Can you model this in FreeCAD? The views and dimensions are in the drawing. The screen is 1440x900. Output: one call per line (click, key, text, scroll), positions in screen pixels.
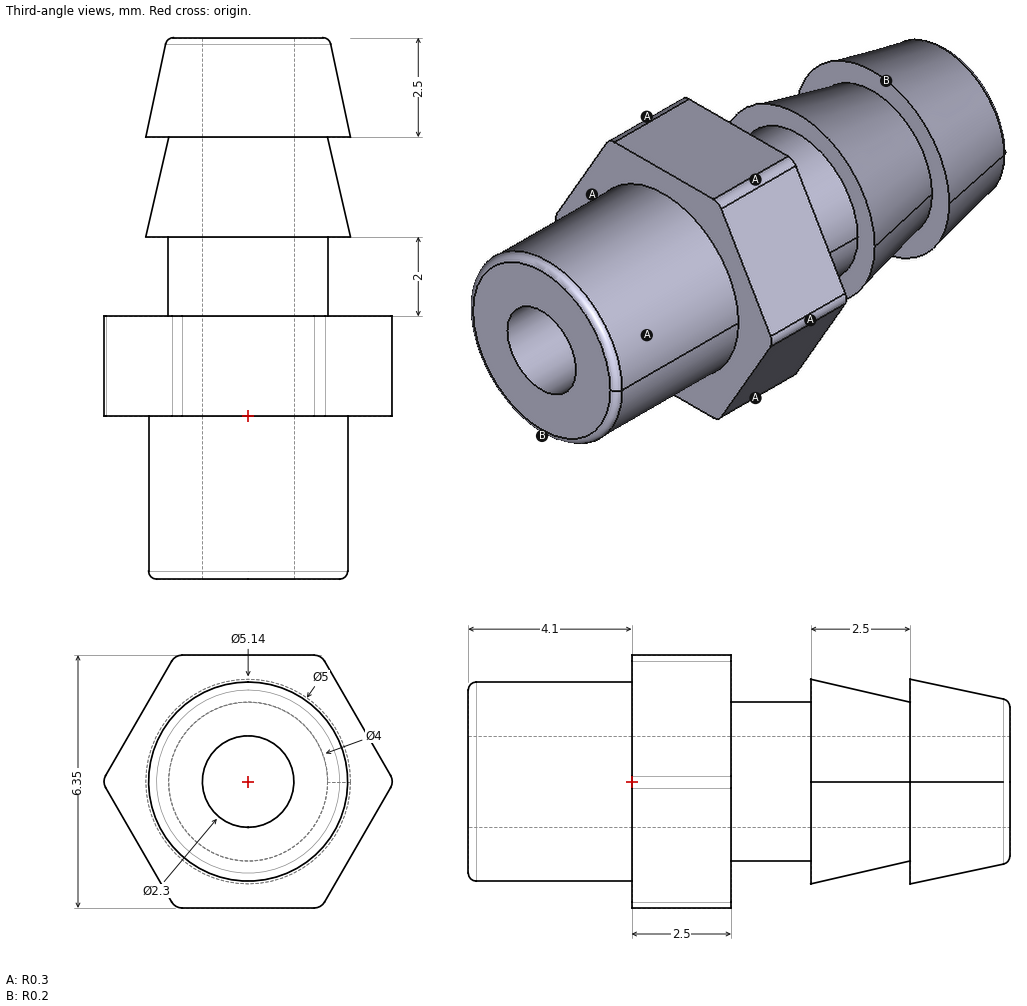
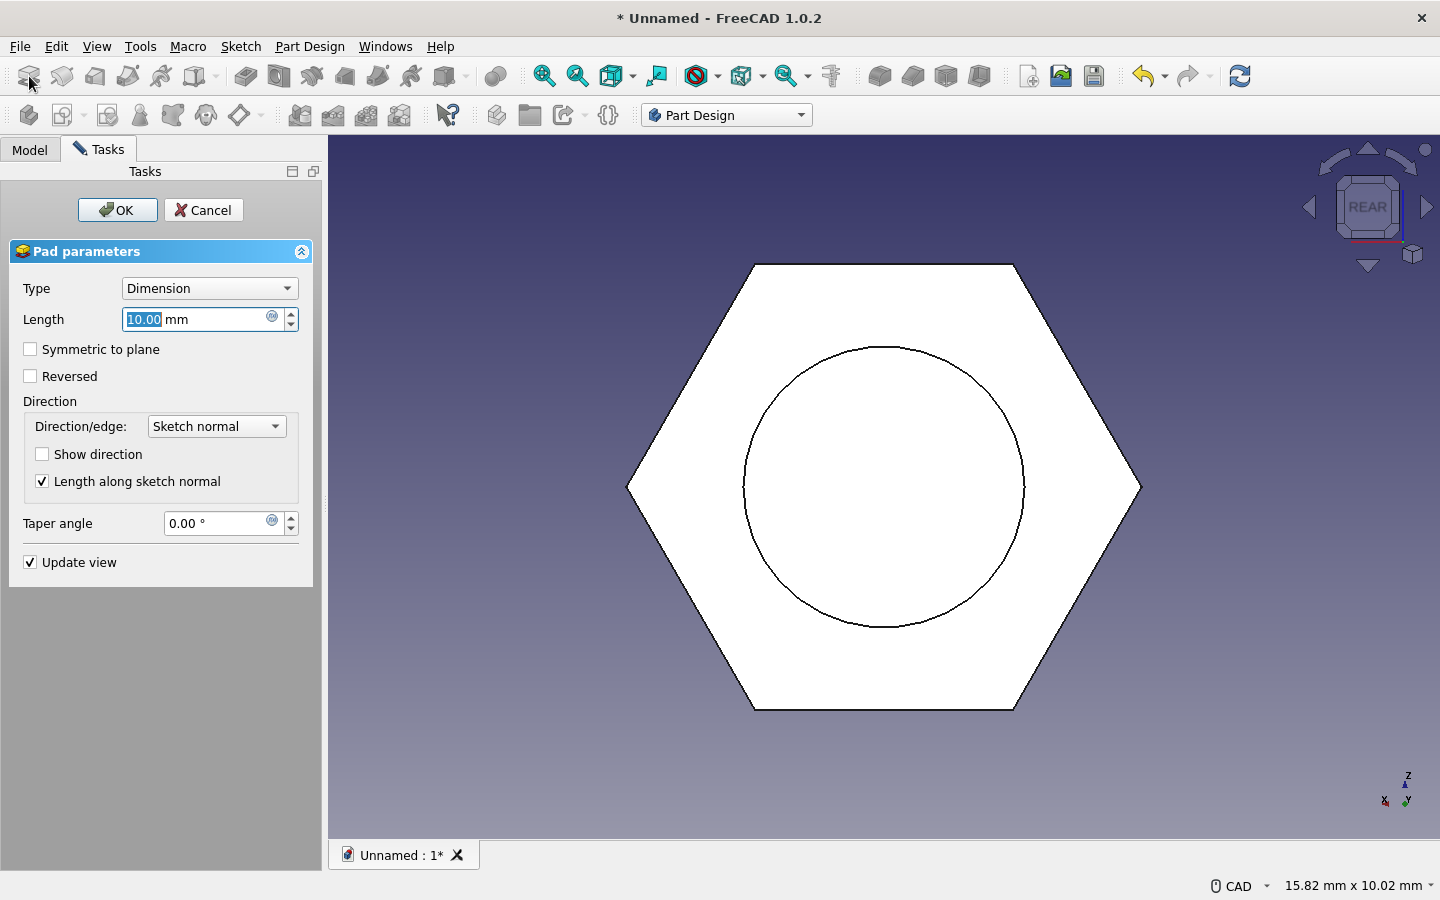
text(2)
key(Tab)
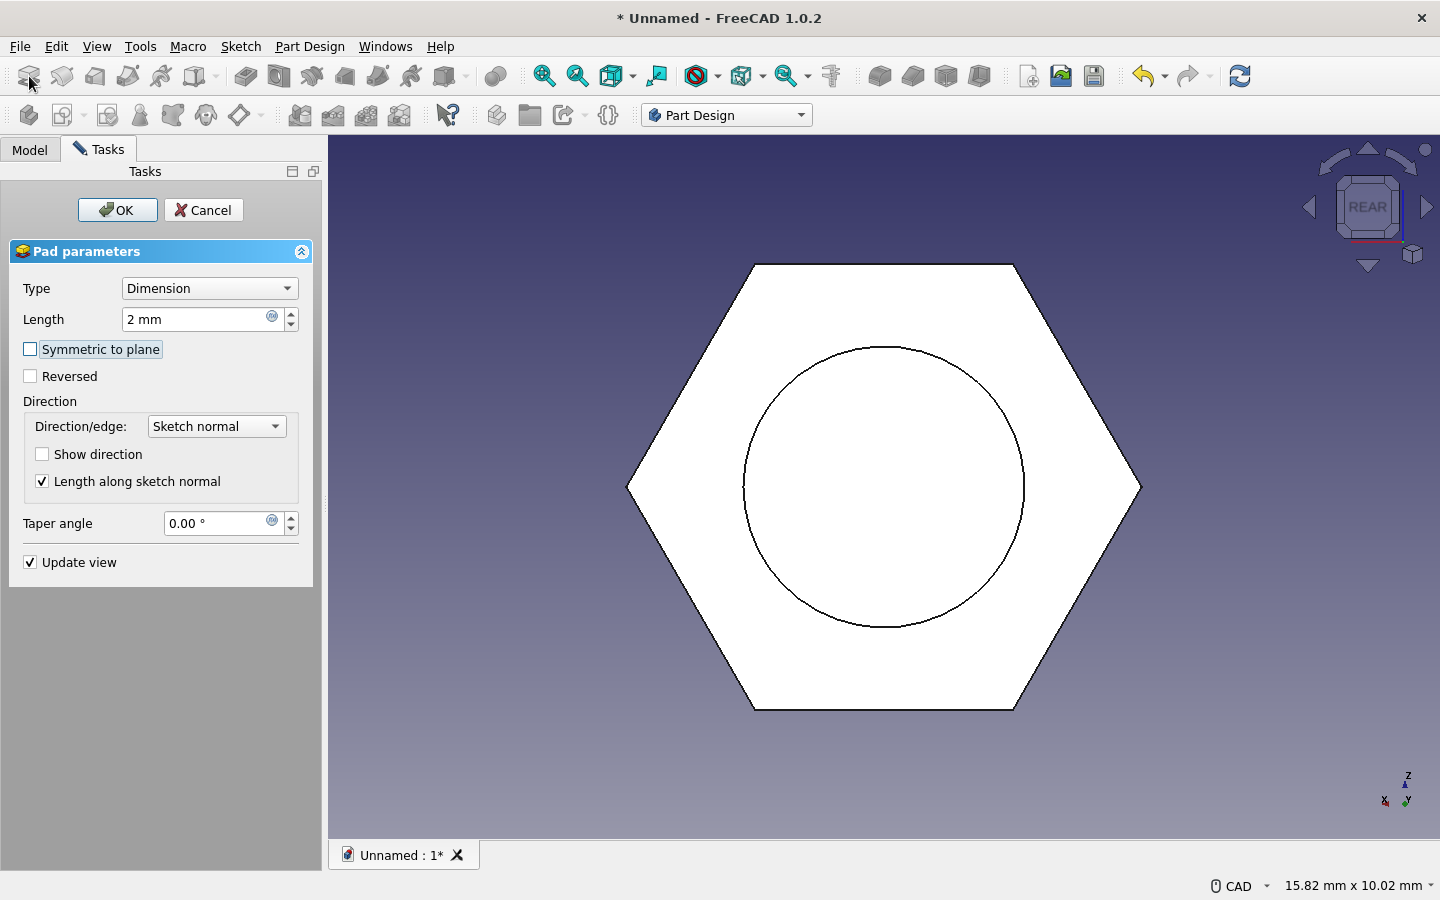
click(118, 210)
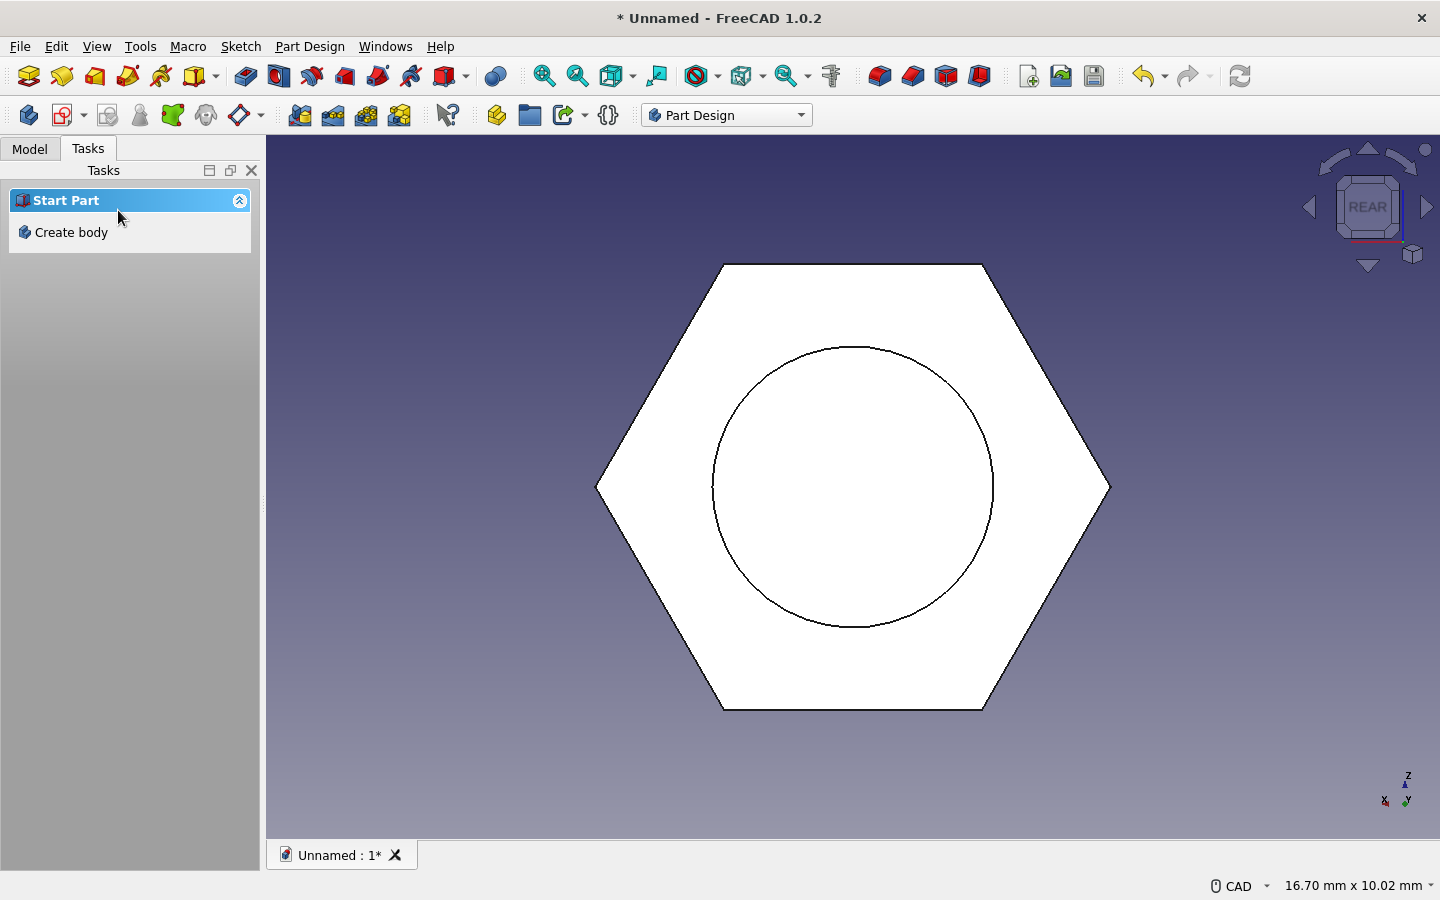
click(853, 486)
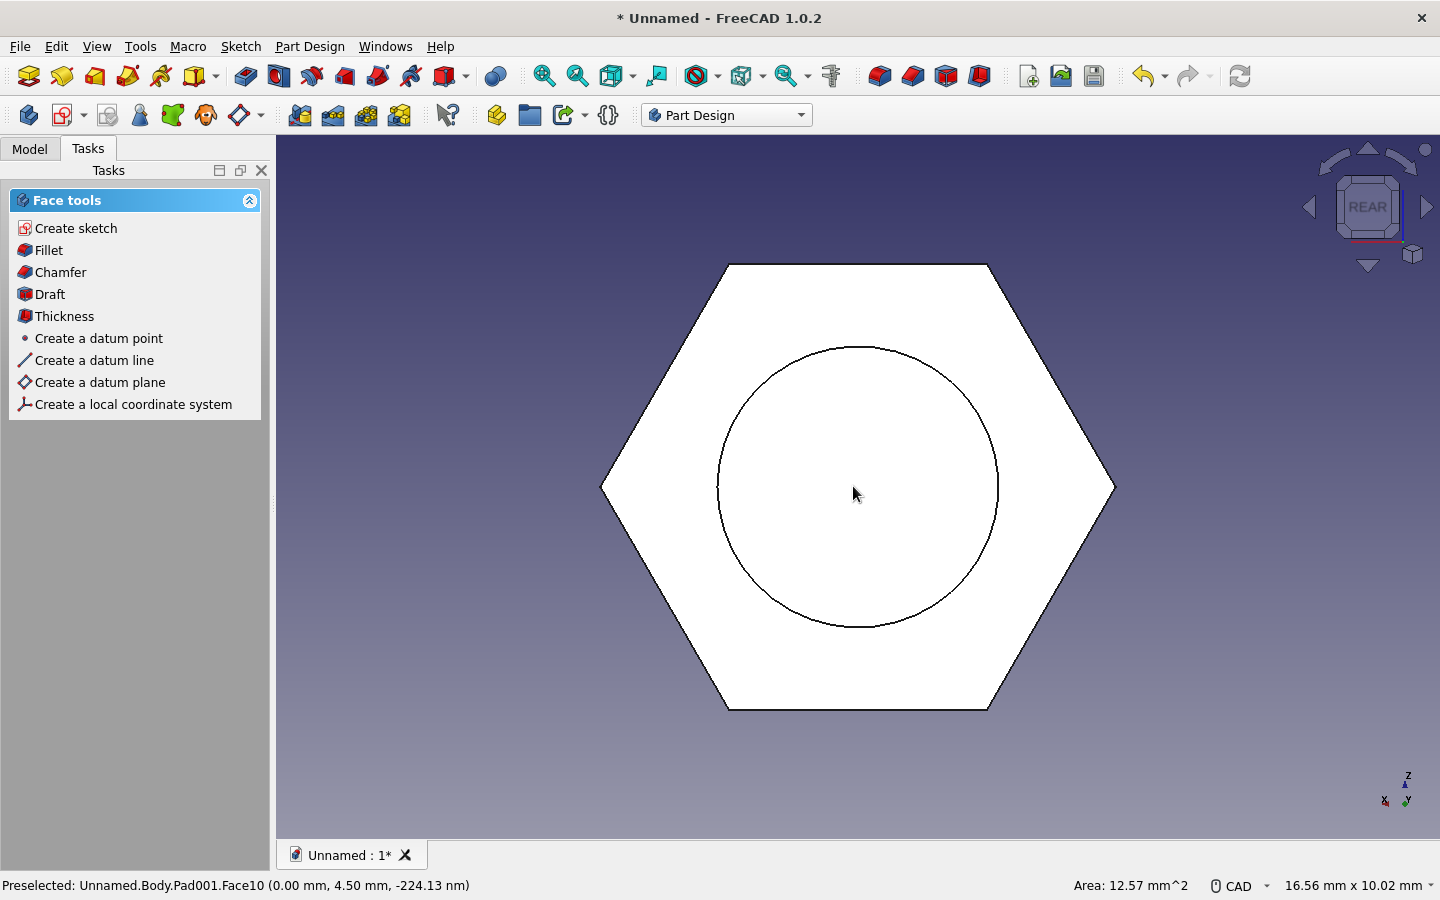
click(62, 116)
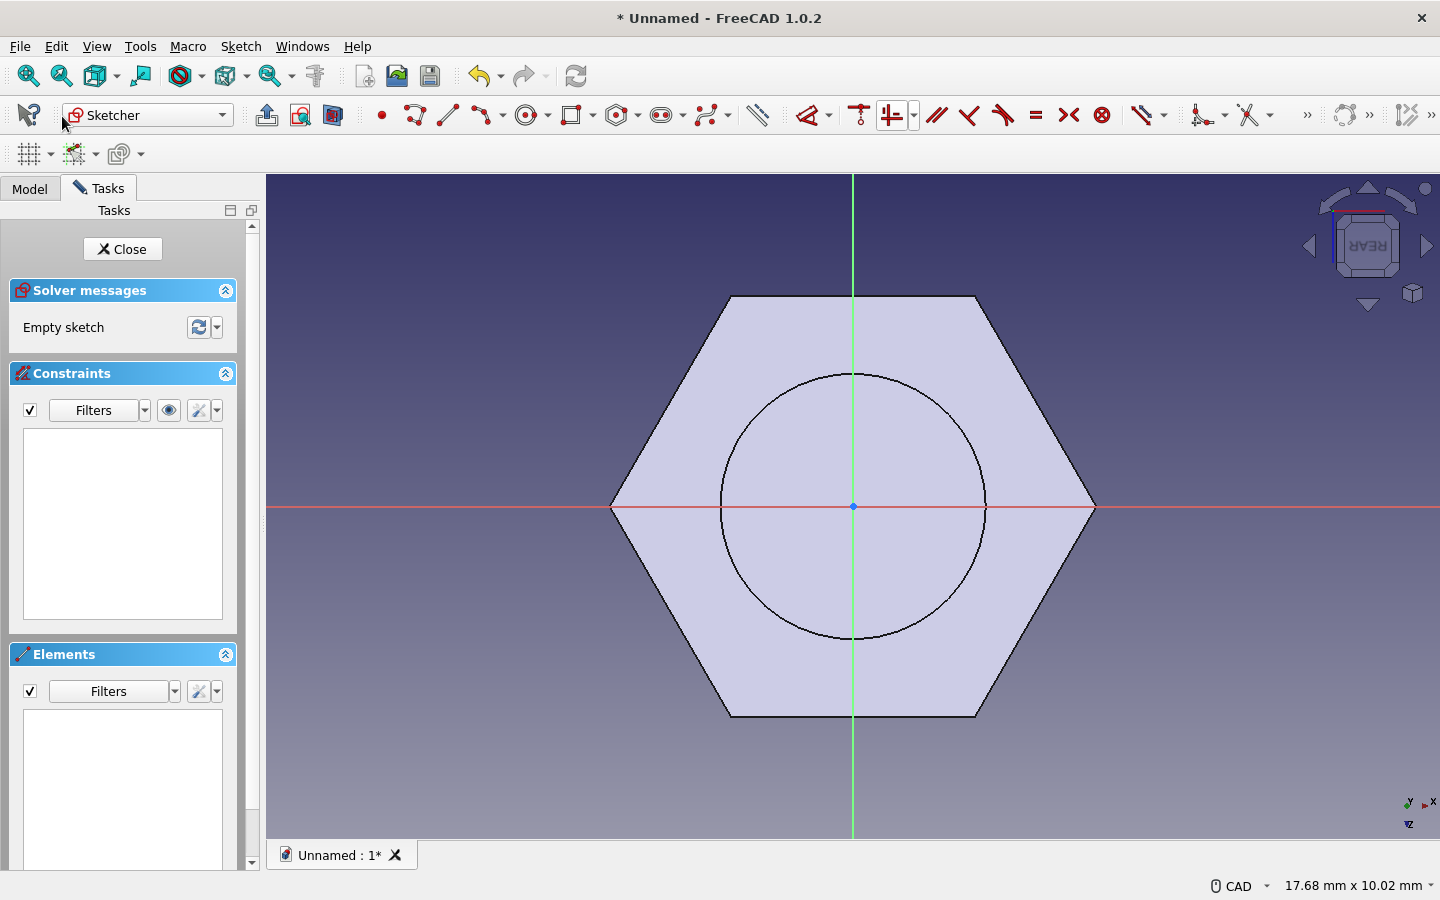
click(526, 116)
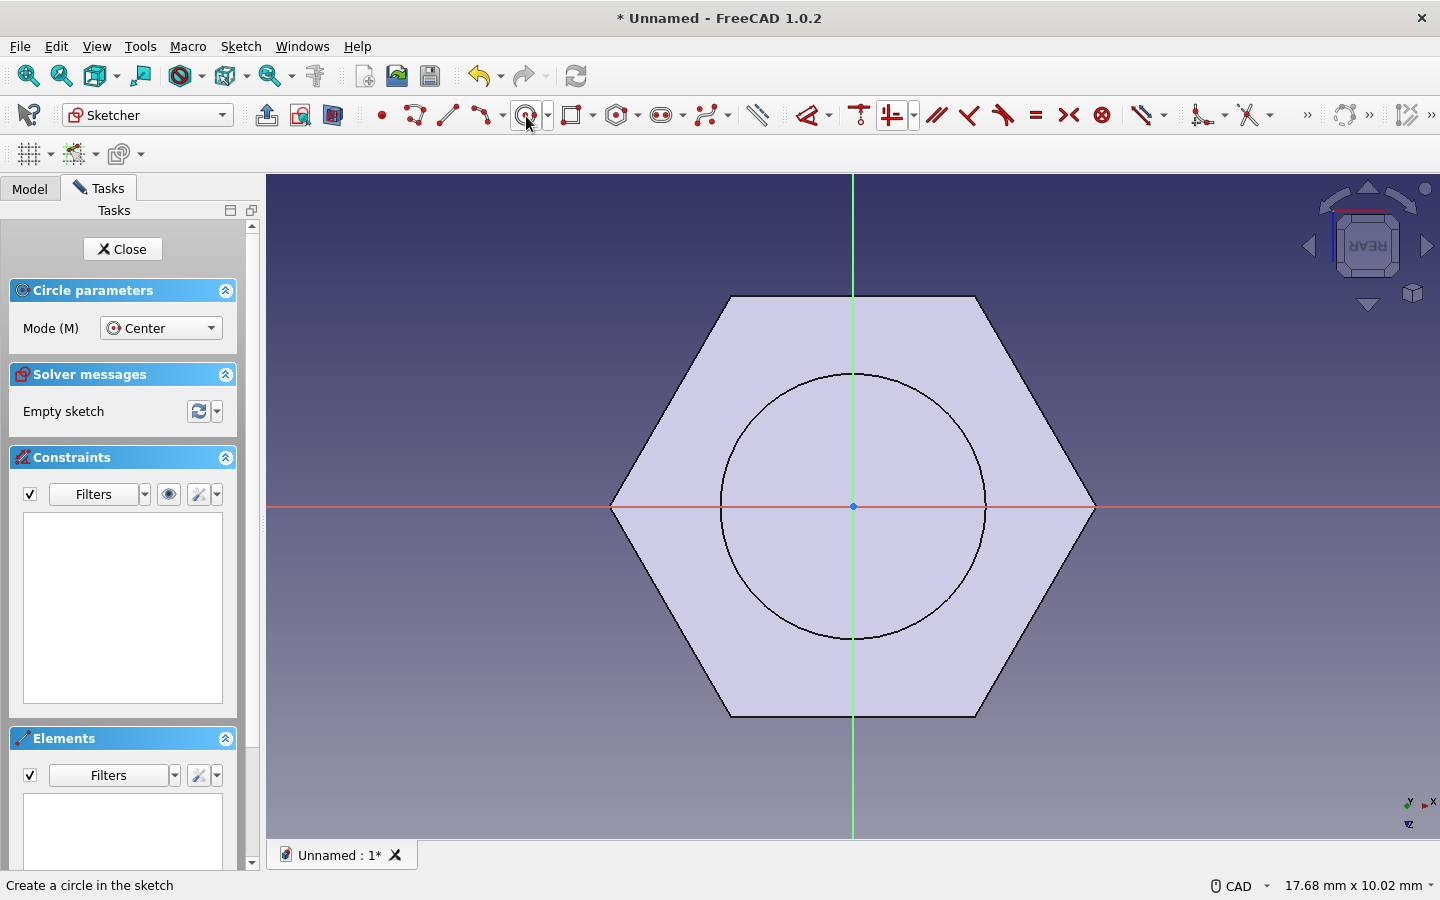
click(853, 507)
click(974, 386)
key(Escape)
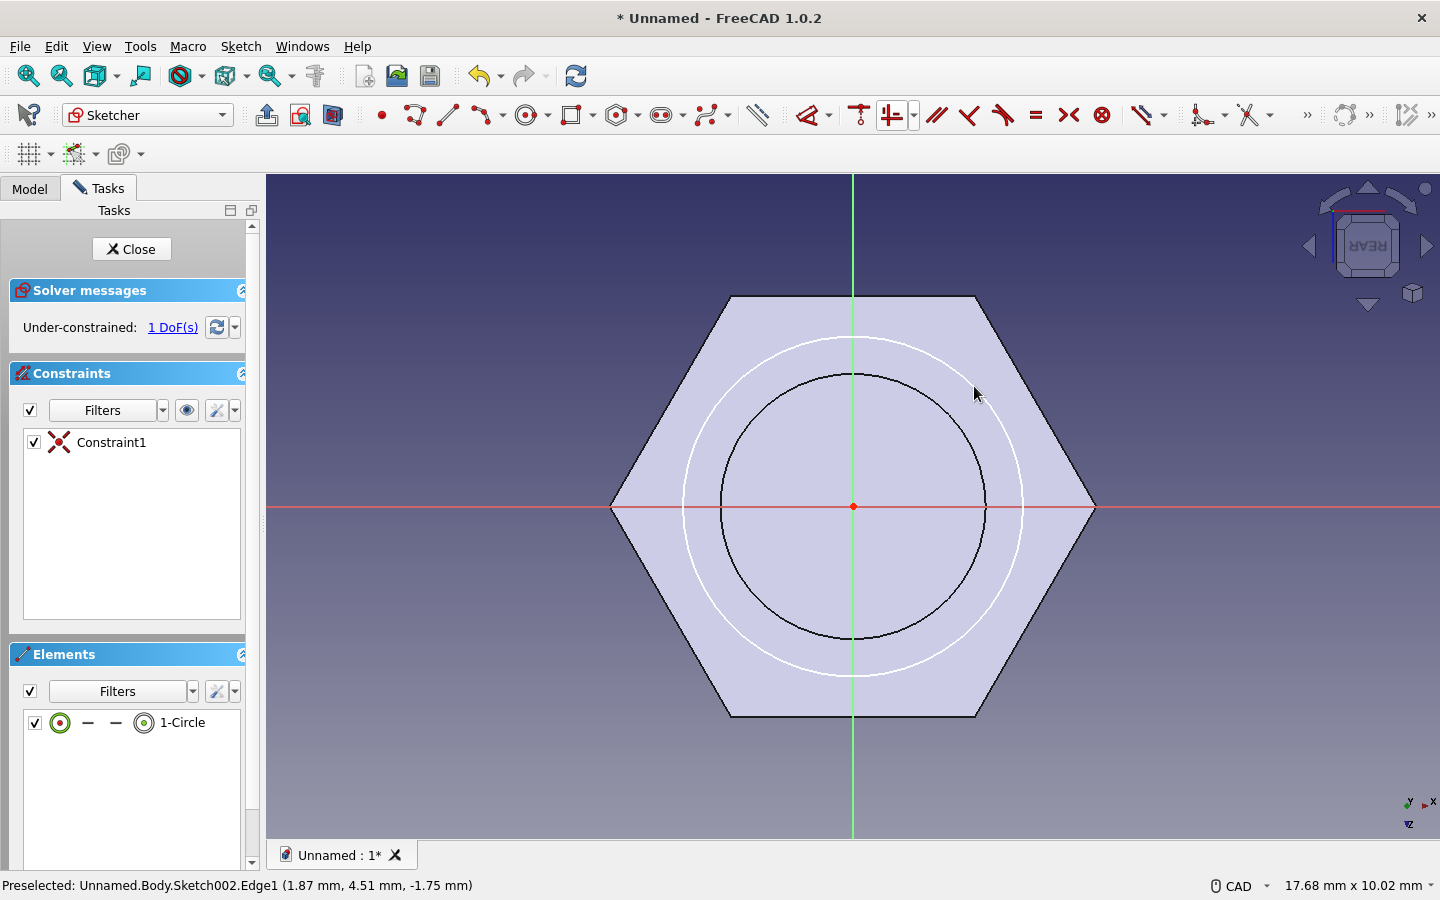
click(806, 116)